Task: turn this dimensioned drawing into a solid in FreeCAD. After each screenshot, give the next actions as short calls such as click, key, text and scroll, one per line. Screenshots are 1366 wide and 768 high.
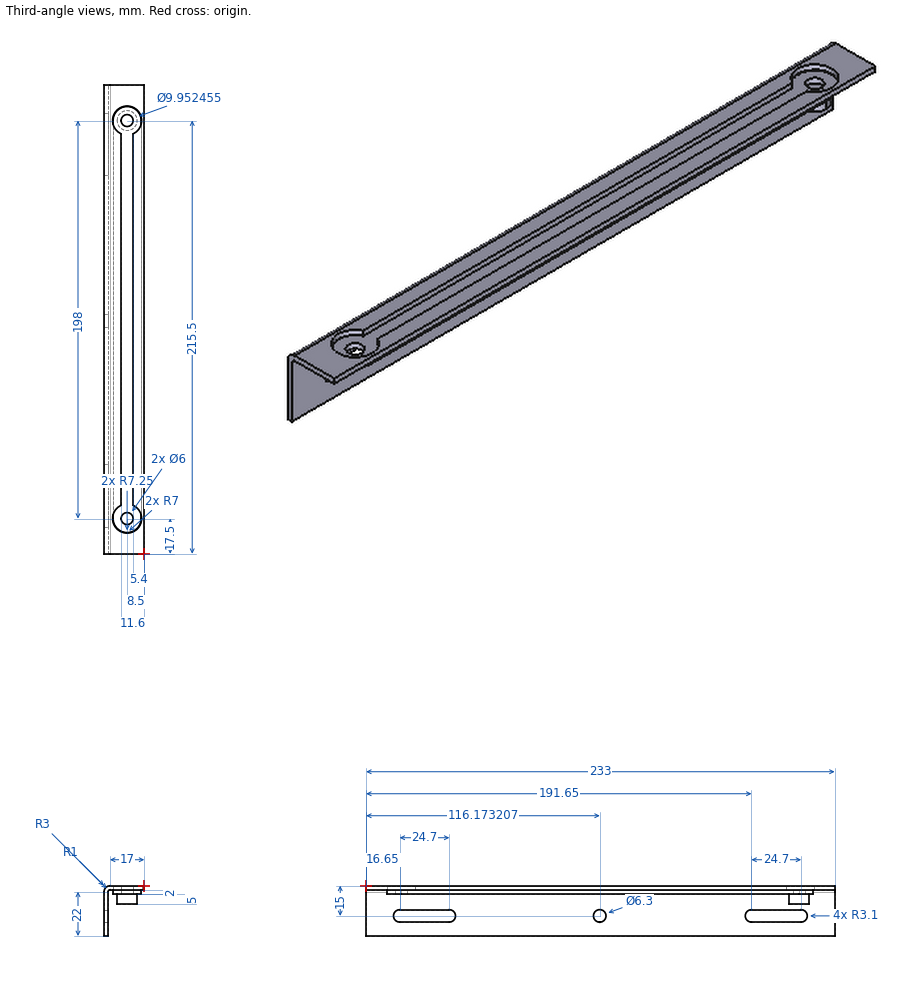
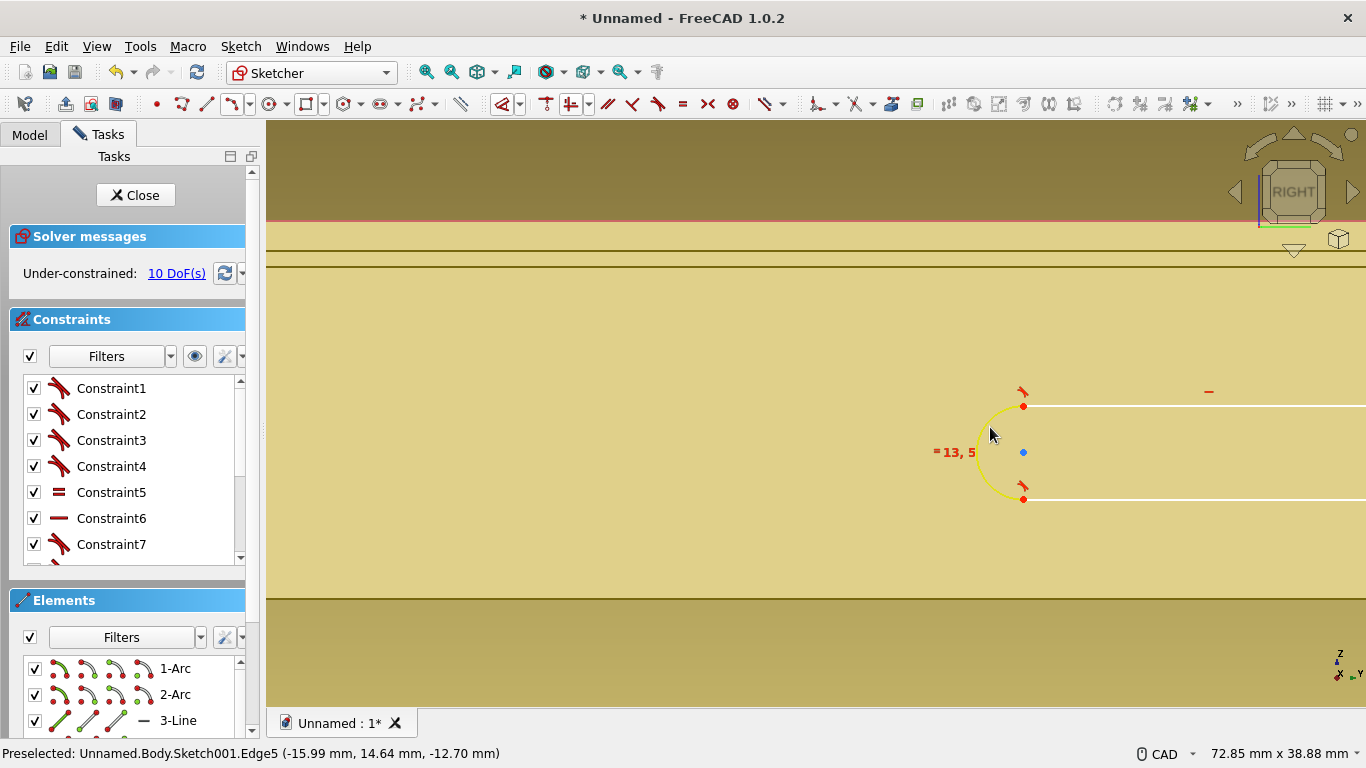
click(986, 425)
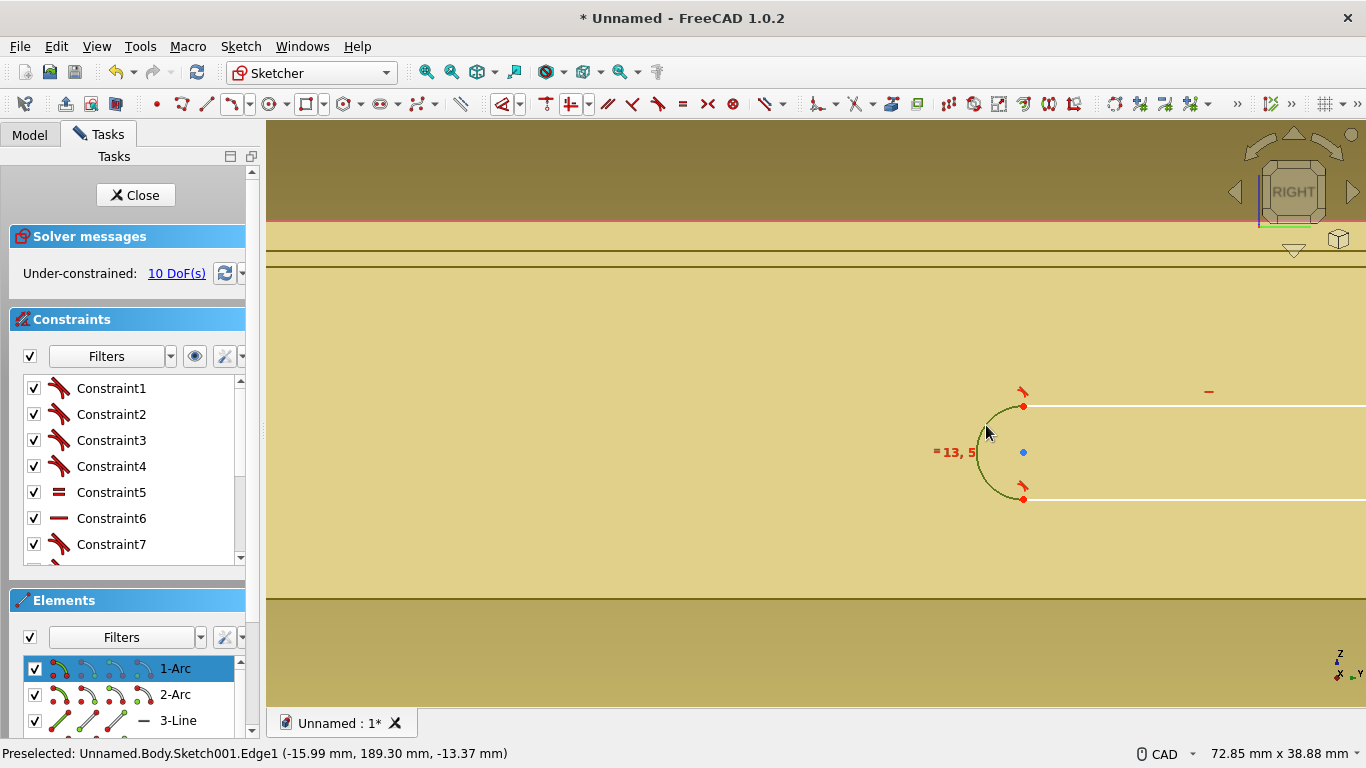
key(k)
key(r)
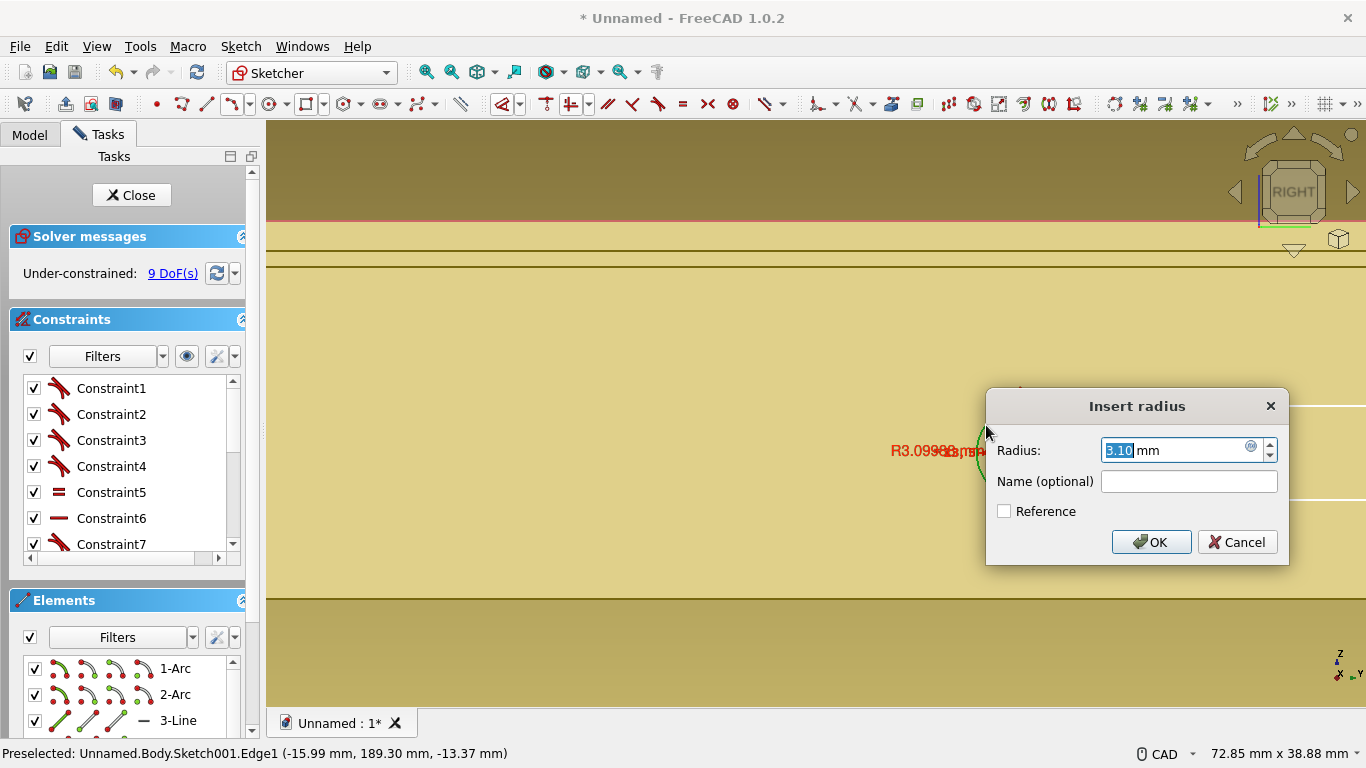
text(3.1)
key(Return)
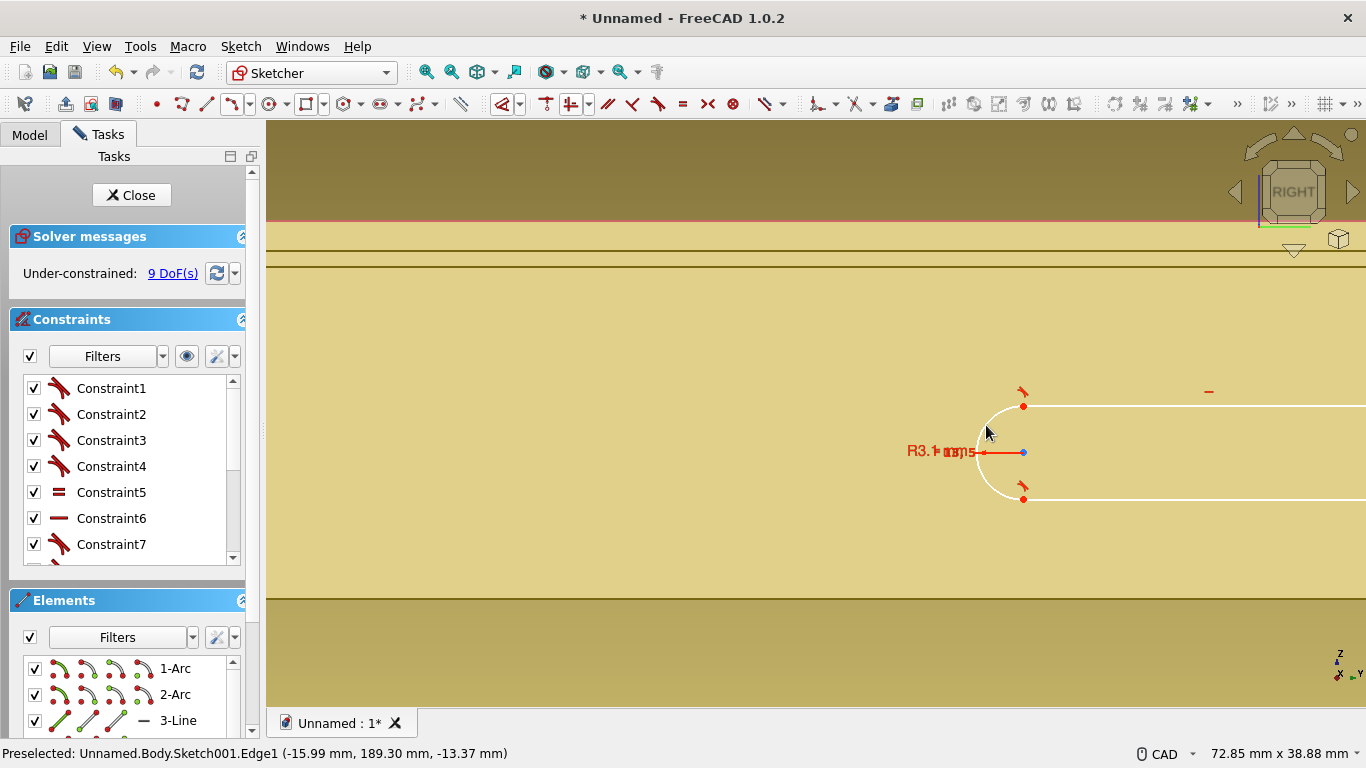
scroll(991, 427, down, 8)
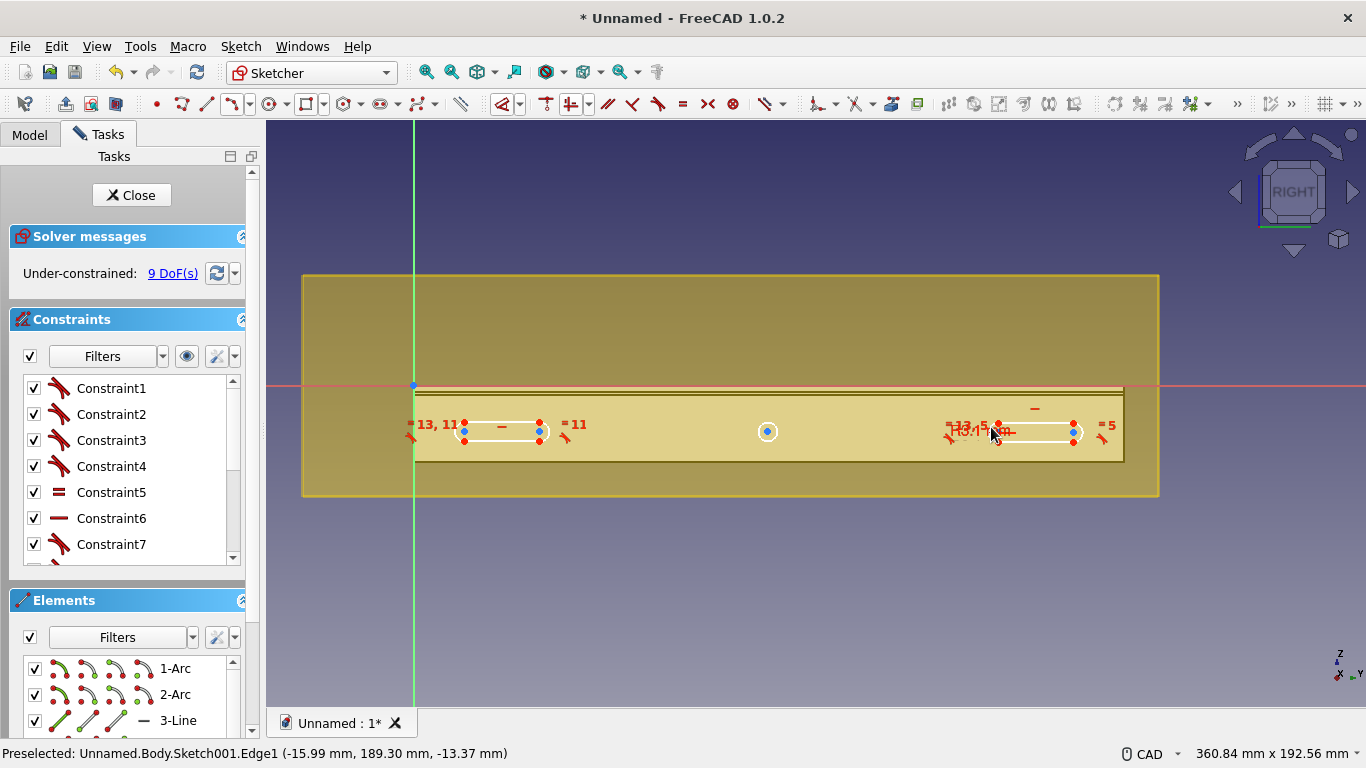
scroll(775, 425, up, 4)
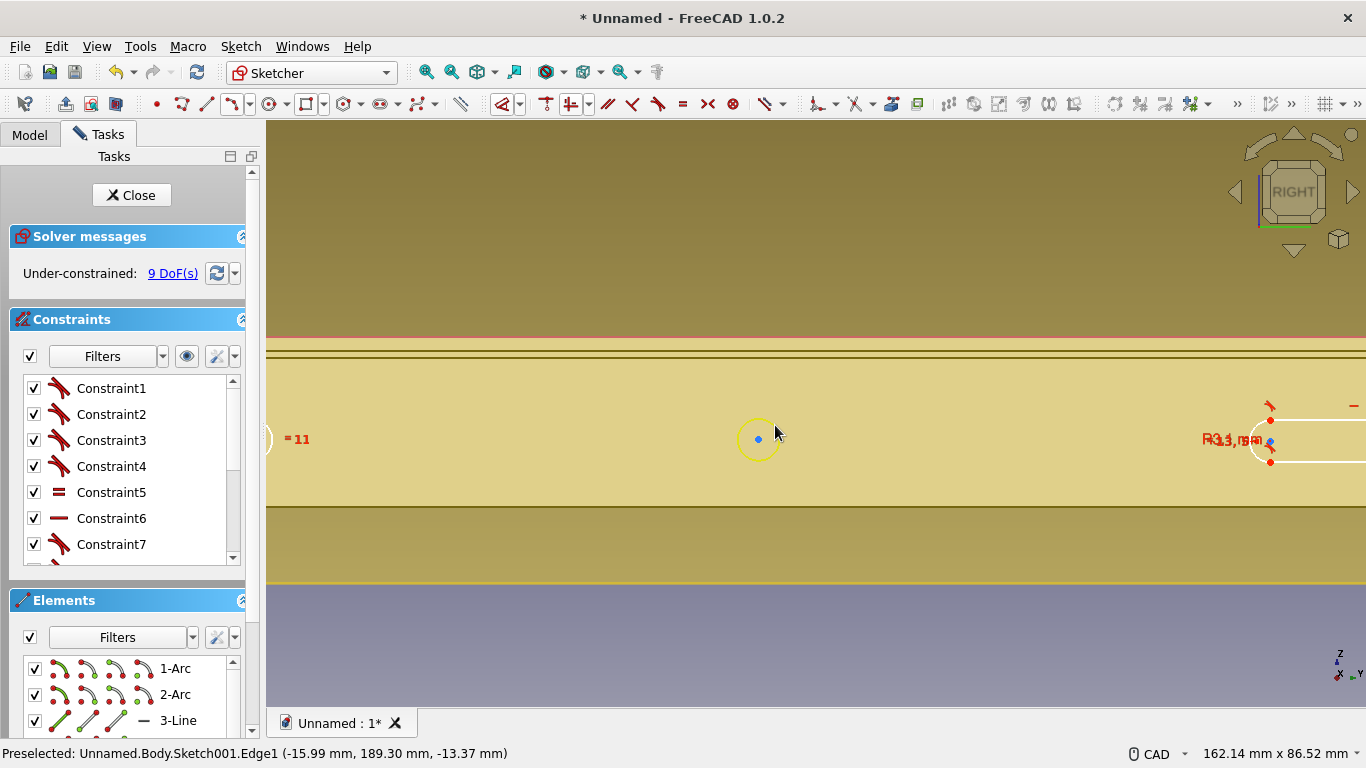
click(773, 425)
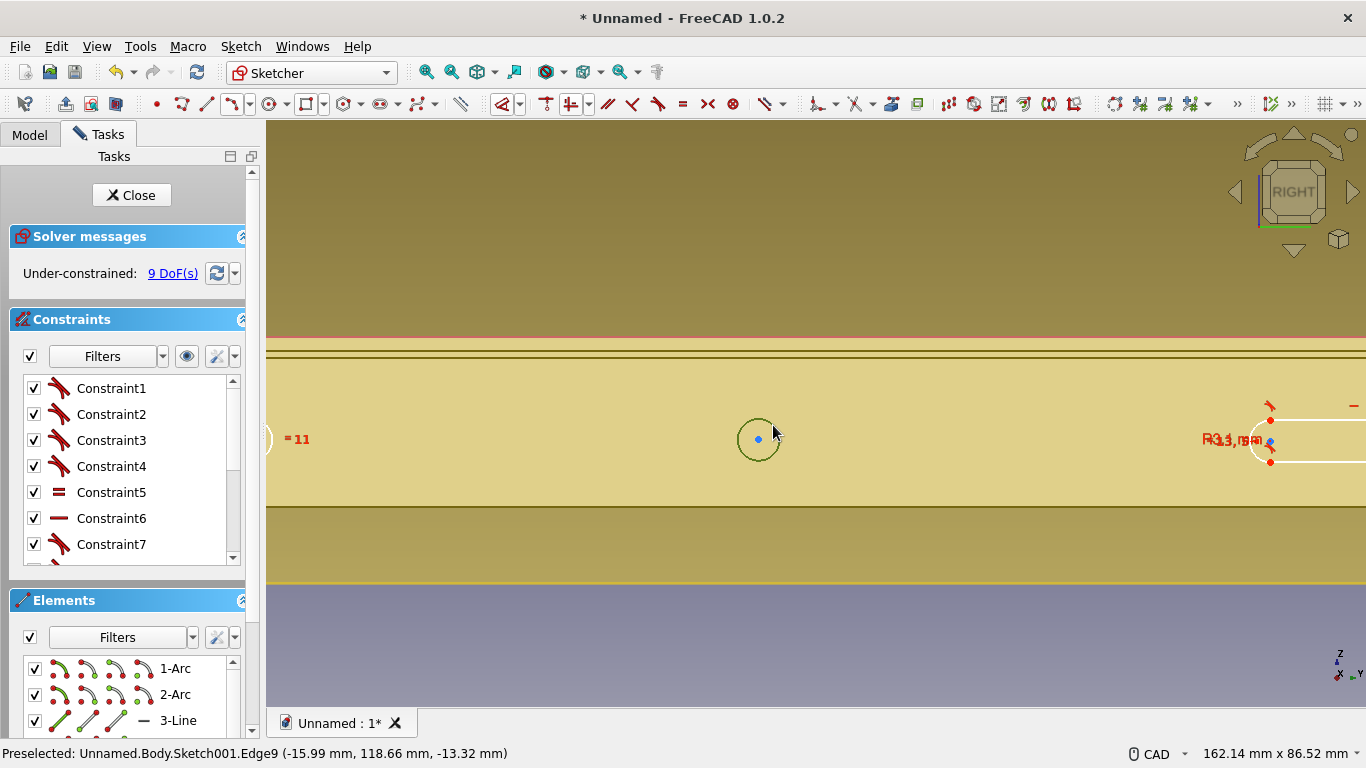
key(k)
key(o)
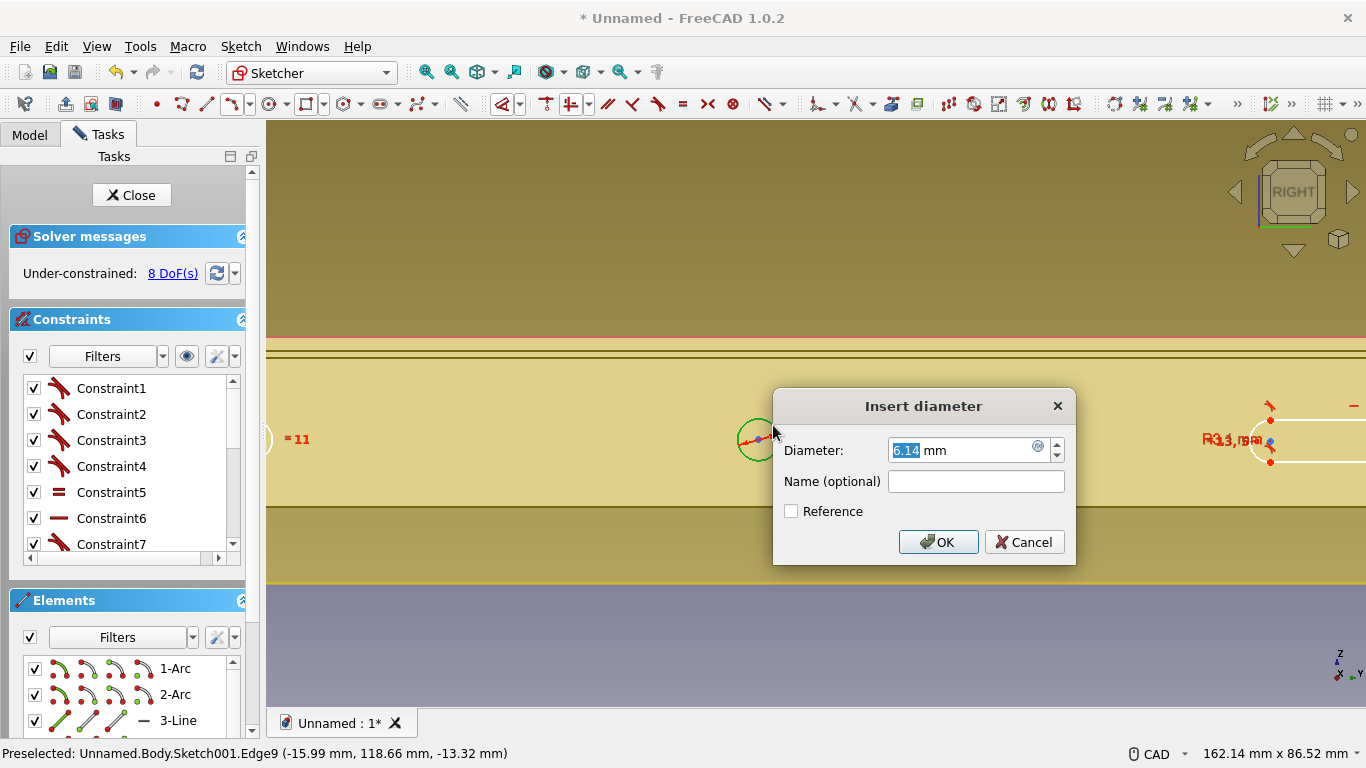
text(6.3)
key(Return)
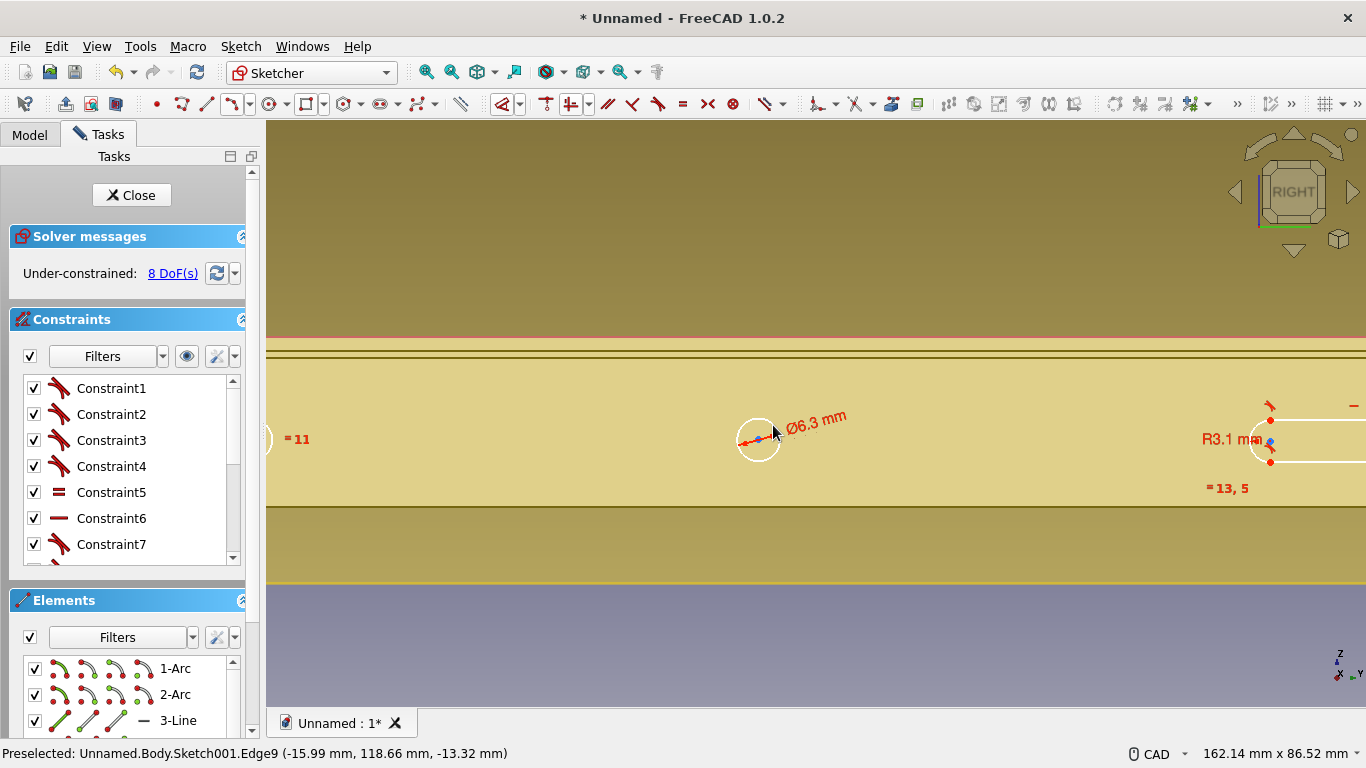
click(759, 440)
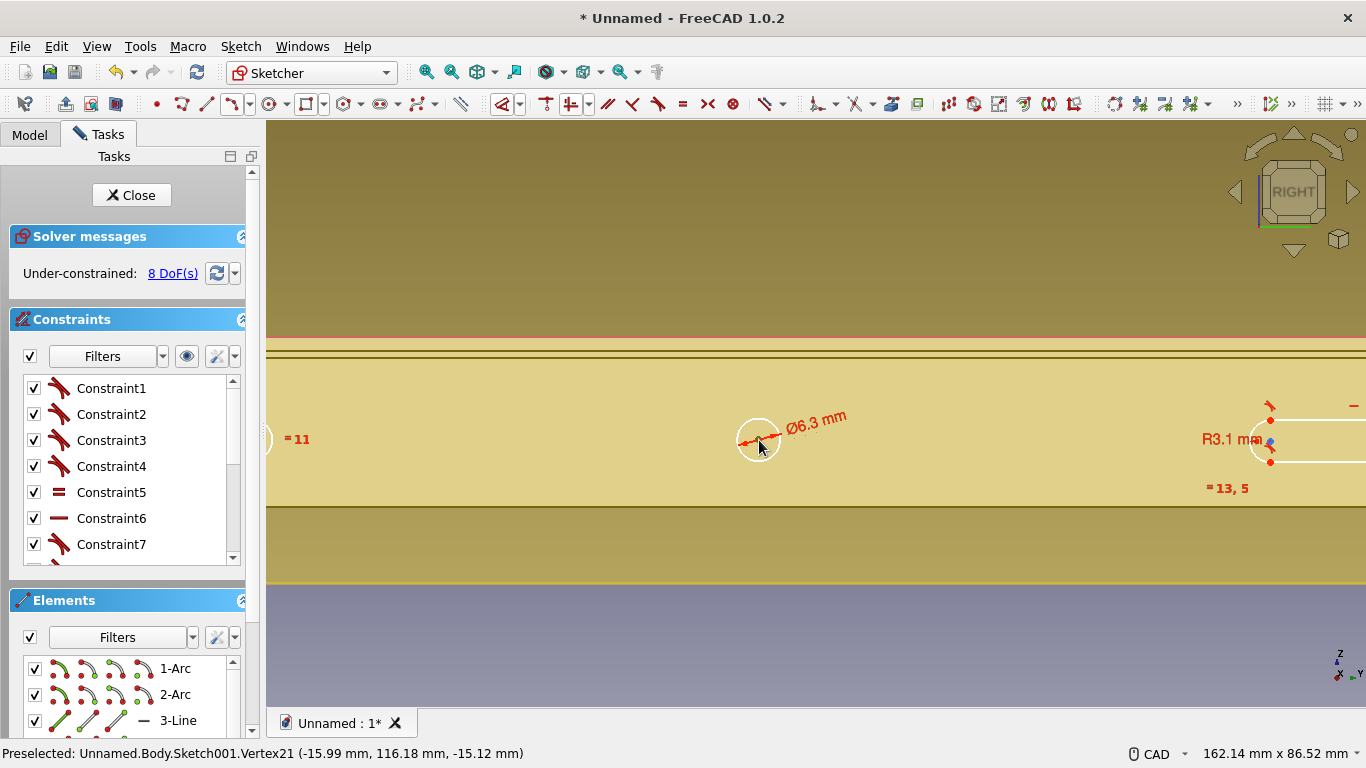
key(i)